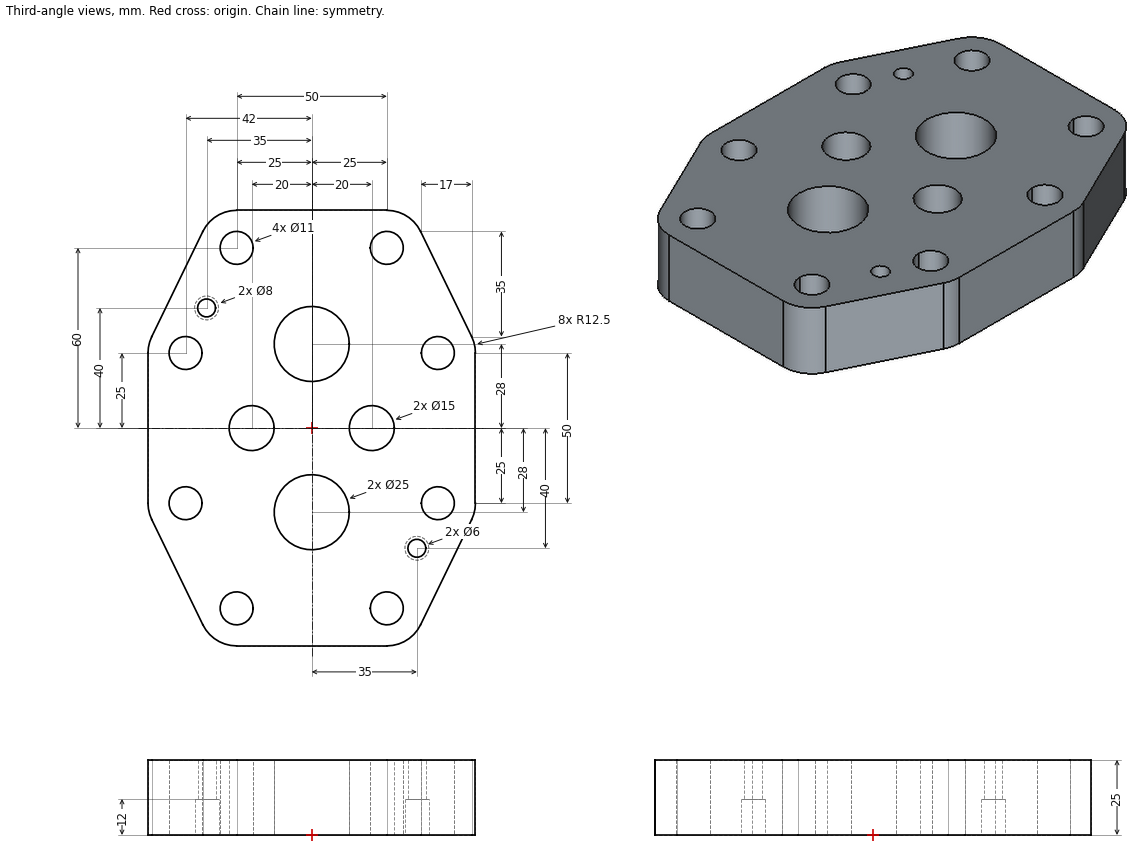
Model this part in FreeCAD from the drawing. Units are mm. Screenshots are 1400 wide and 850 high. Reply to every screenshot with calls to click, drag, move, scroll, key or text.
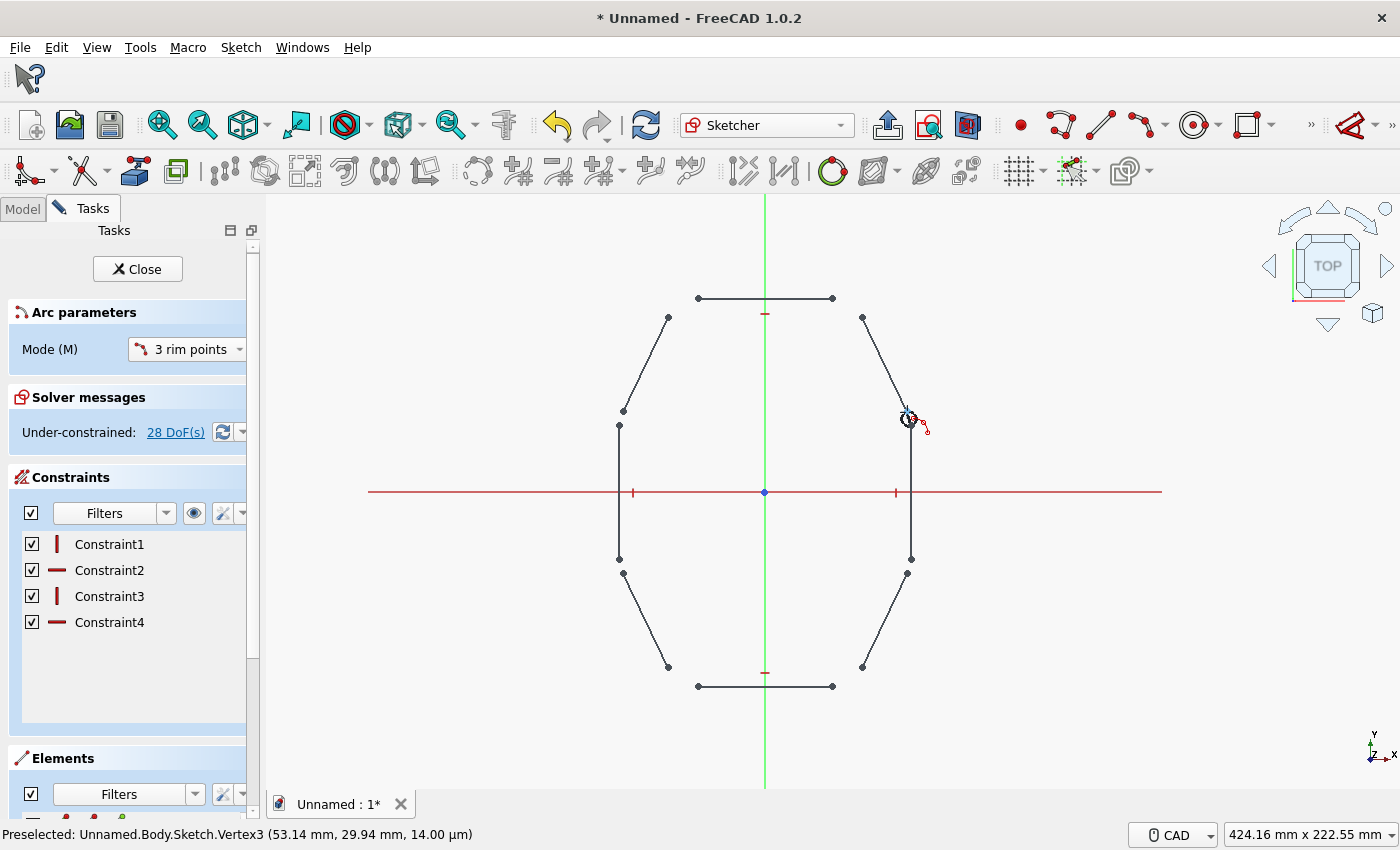
scroll(910, 418, up, 15)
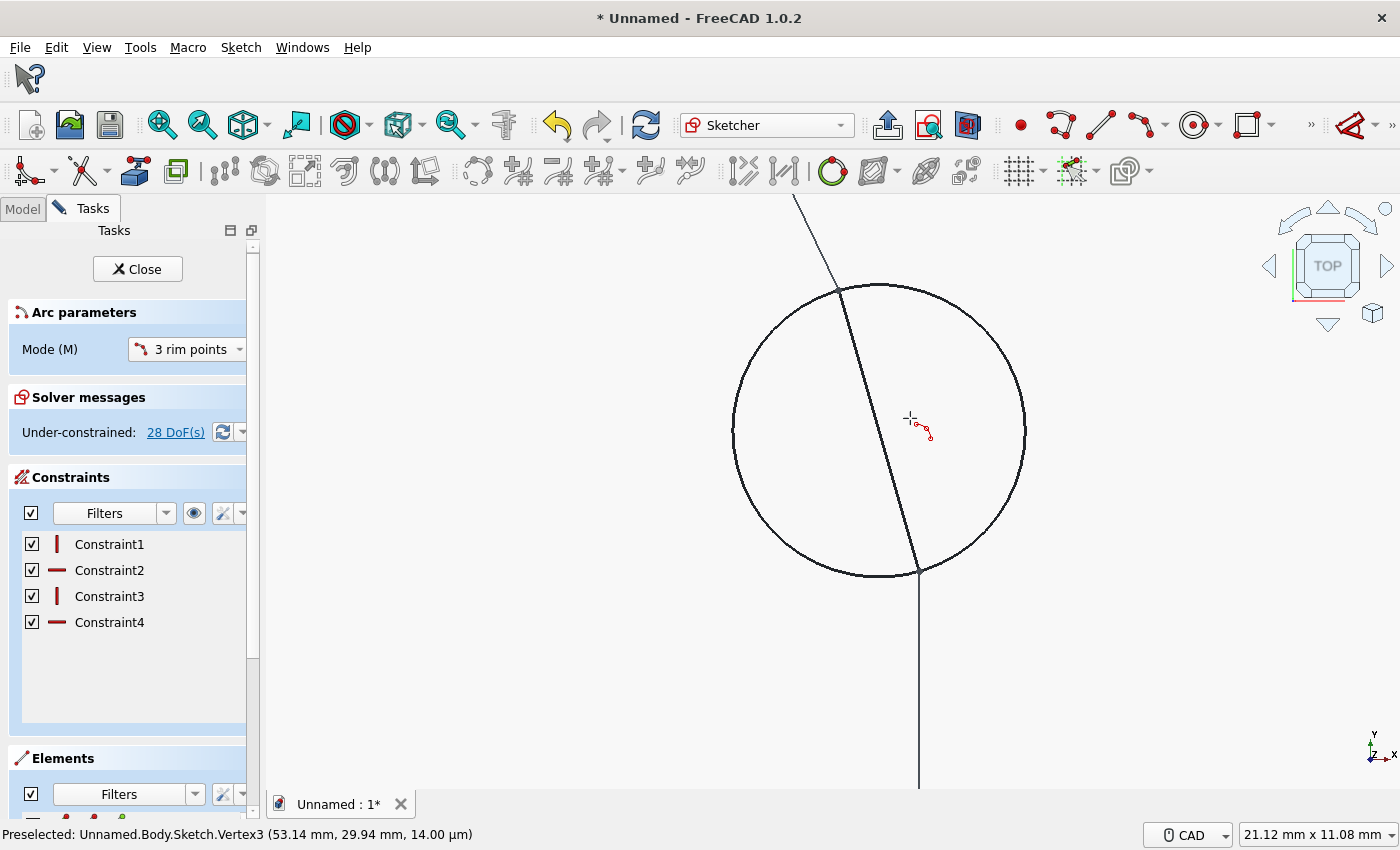
click(895, 405)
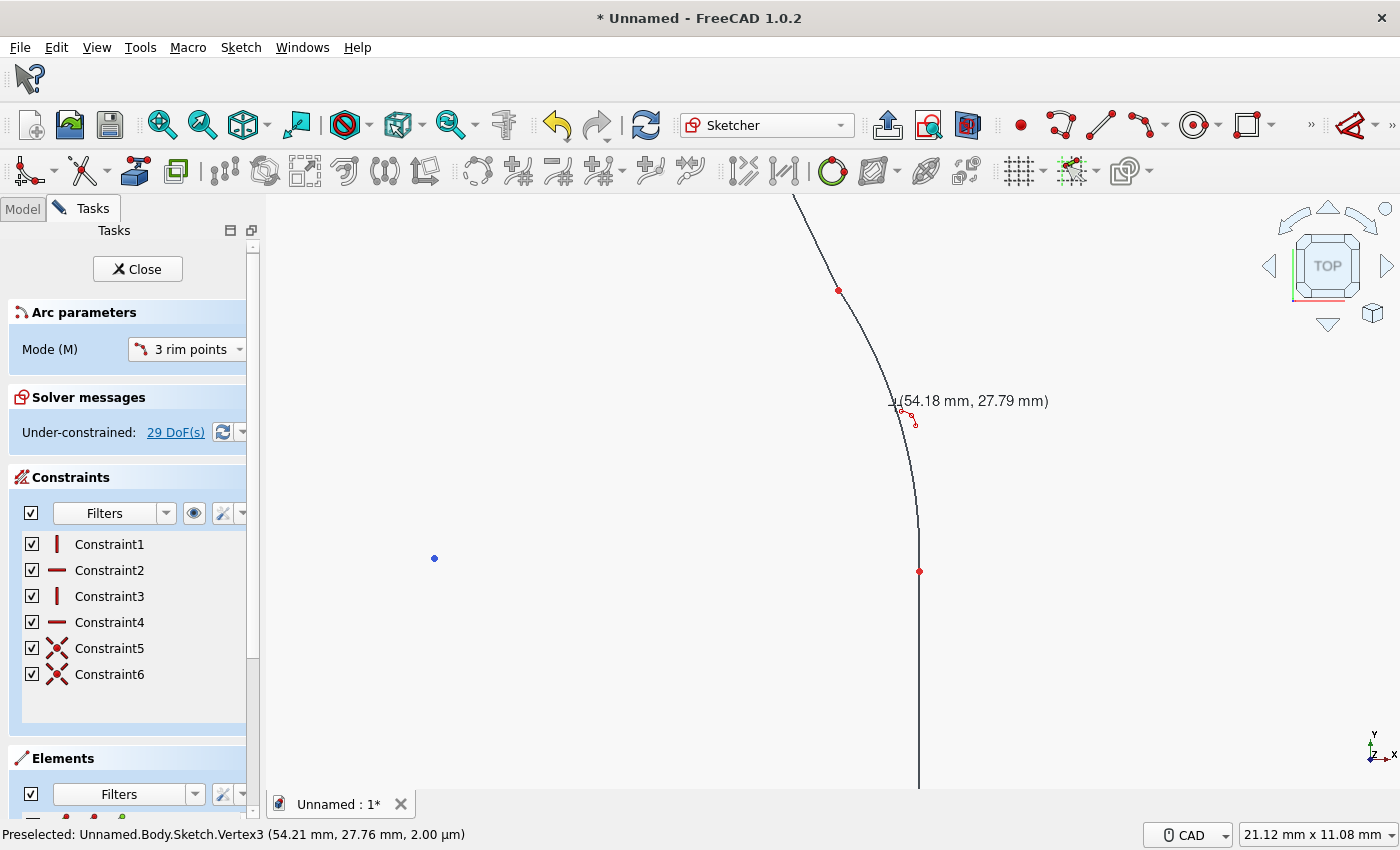
scroll(910, 418, down, 15)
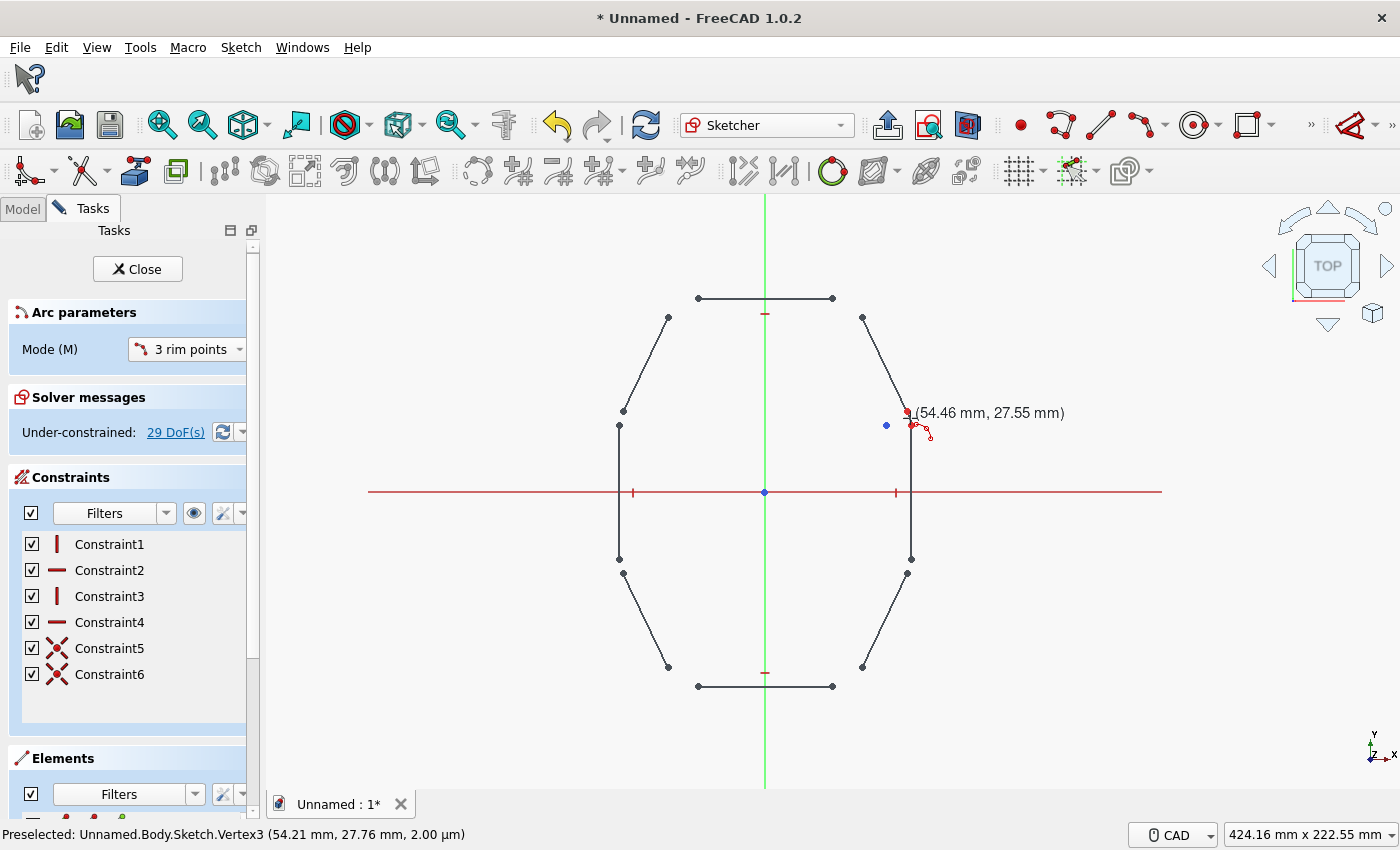
click(862, 318)
click(832, 299)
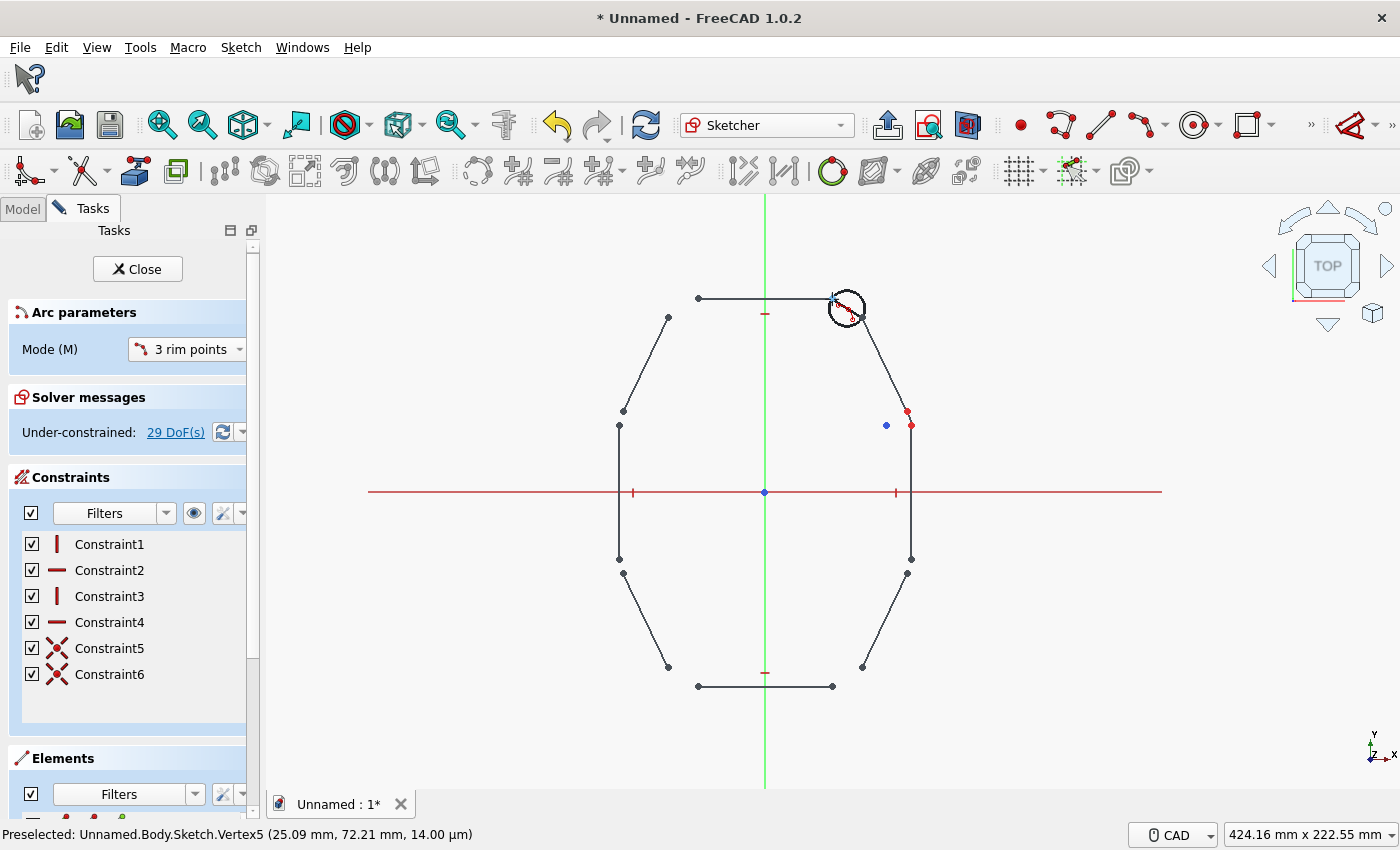
scroll(850, 303, up, 6)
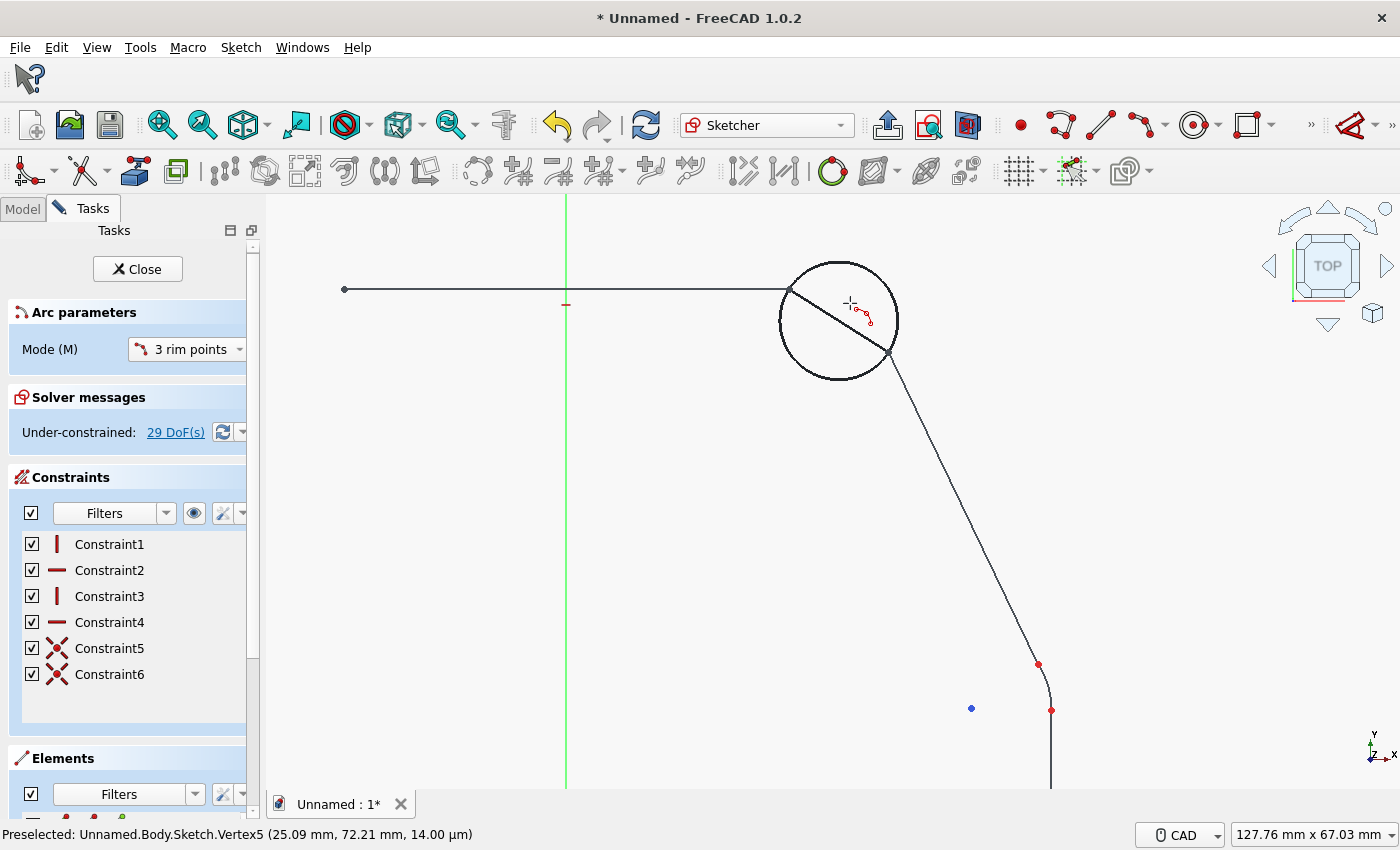
click(847, 304)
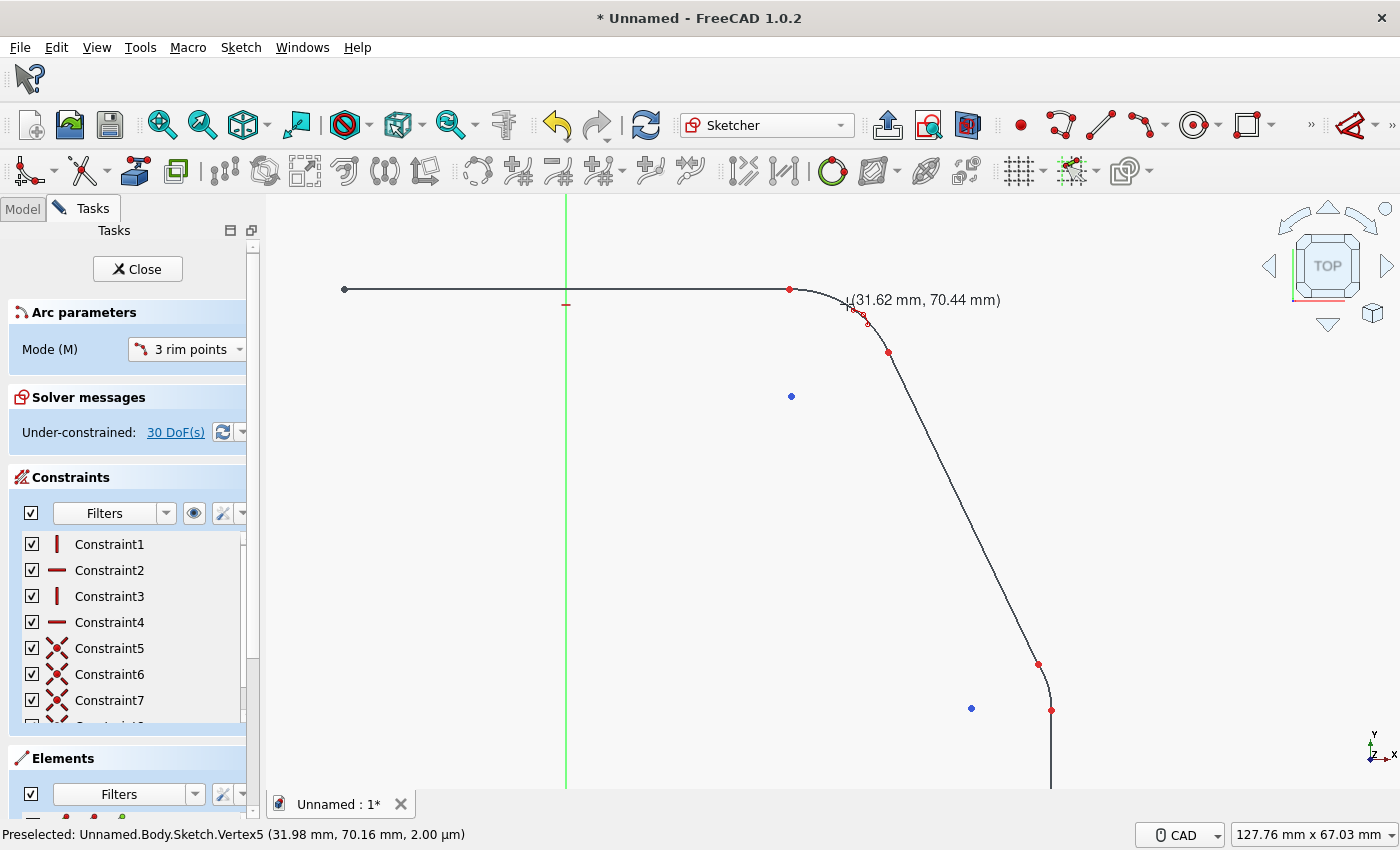
click(344, 289)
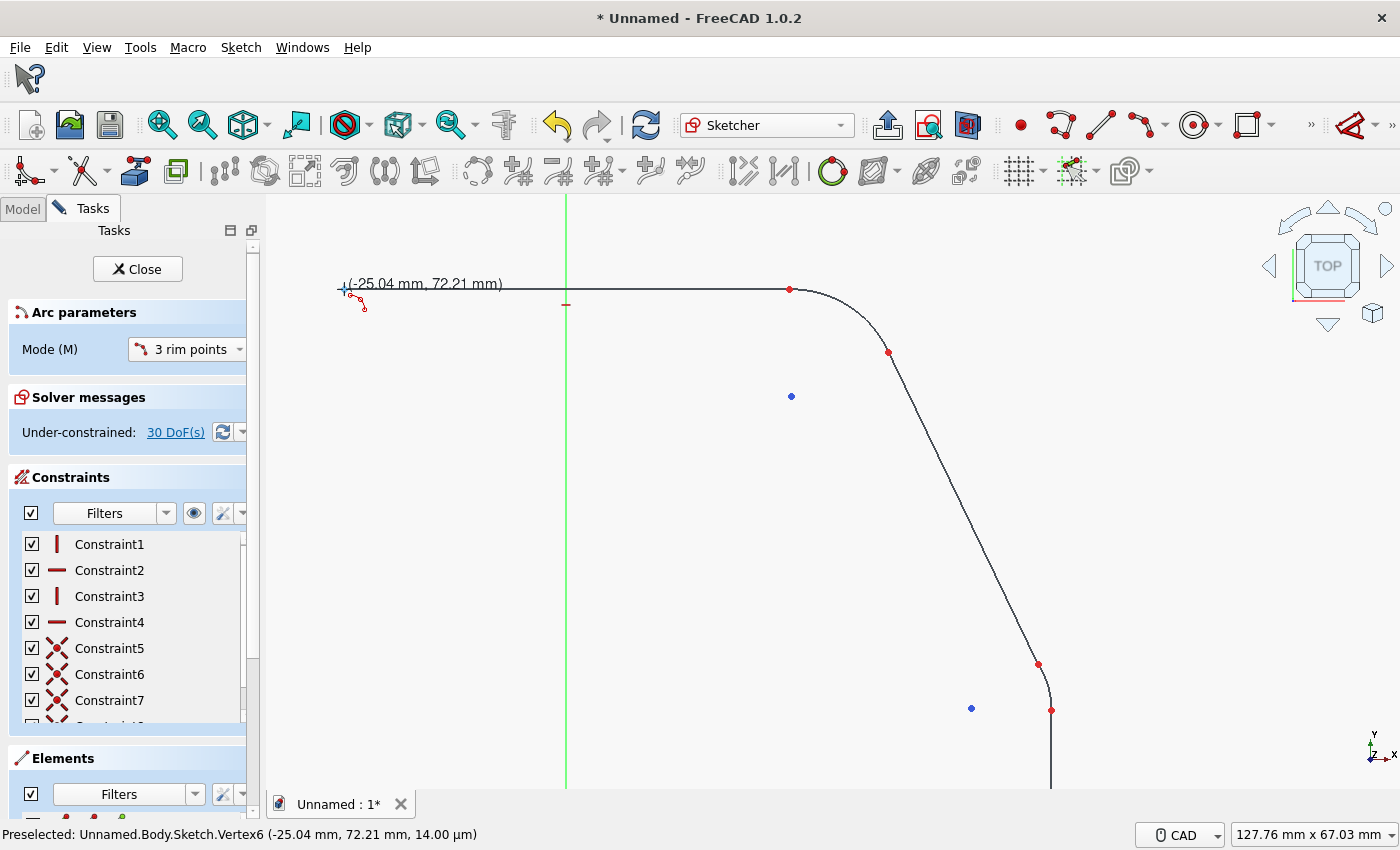
scroll(850, 302, down, 6)